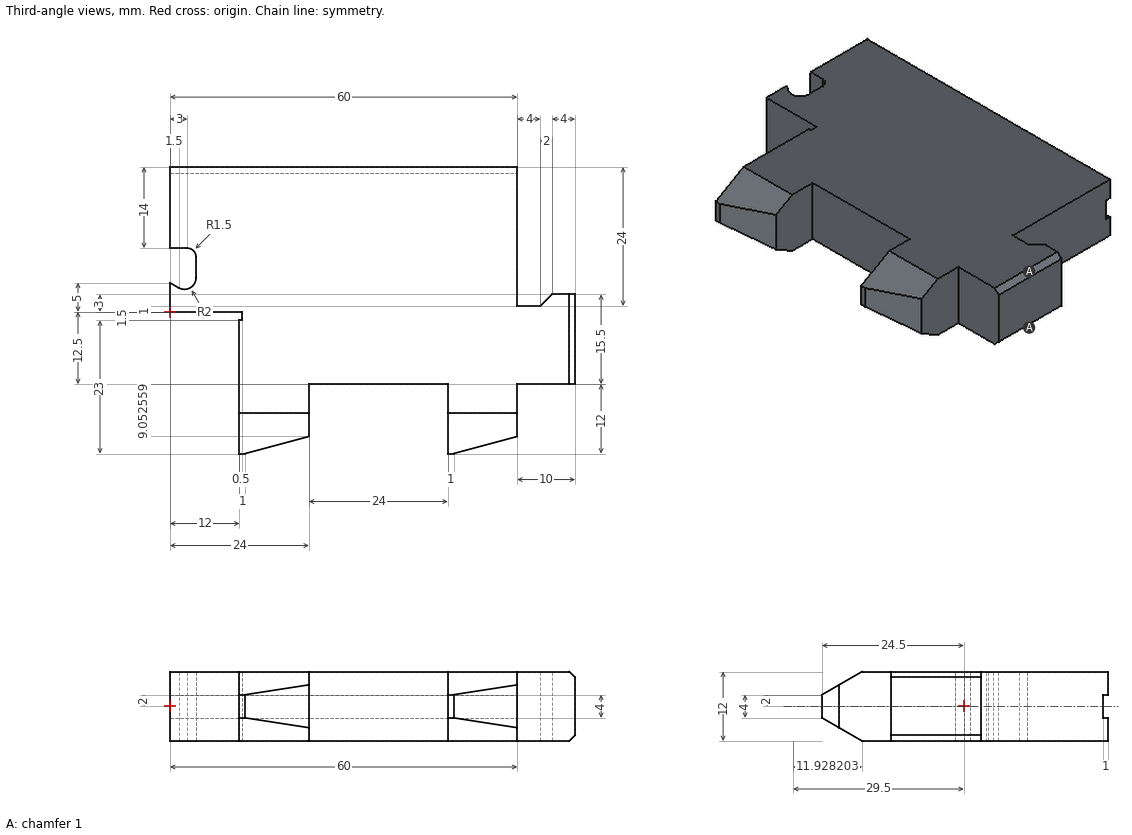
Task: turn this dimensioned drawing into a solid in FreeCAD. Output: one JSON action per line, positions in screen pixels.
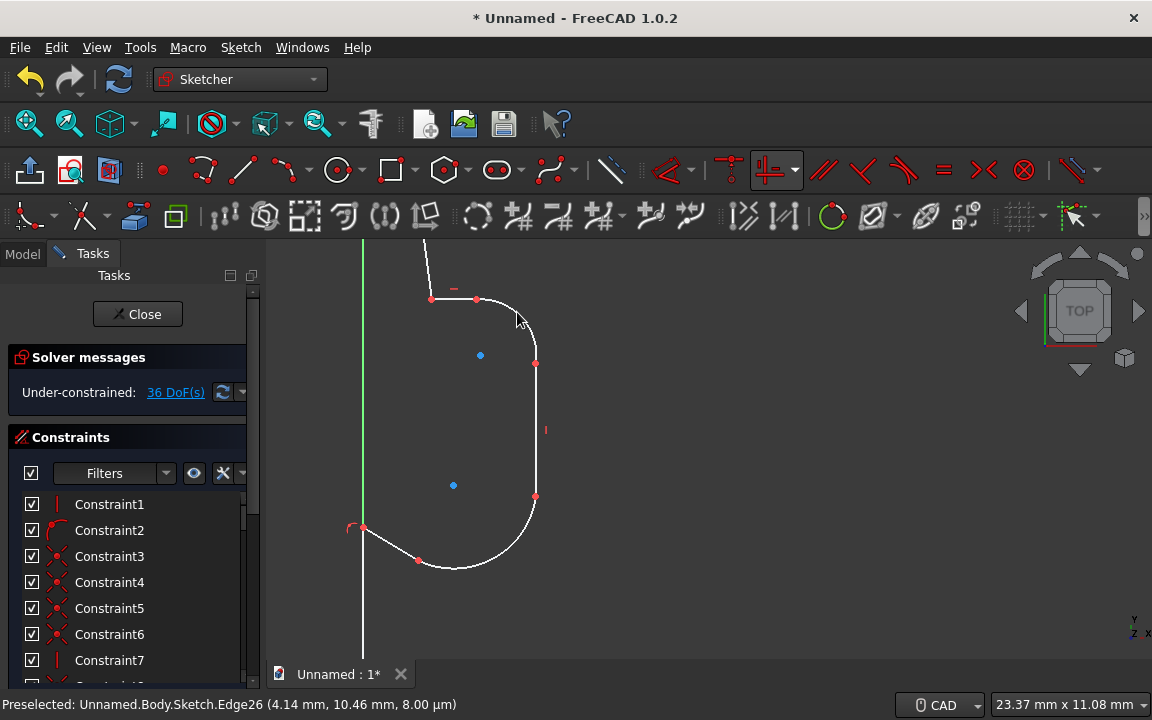
{"action": "scroll", "coordinate": [476, 409], "scroll_direction": "down", "scroll_amount": 10}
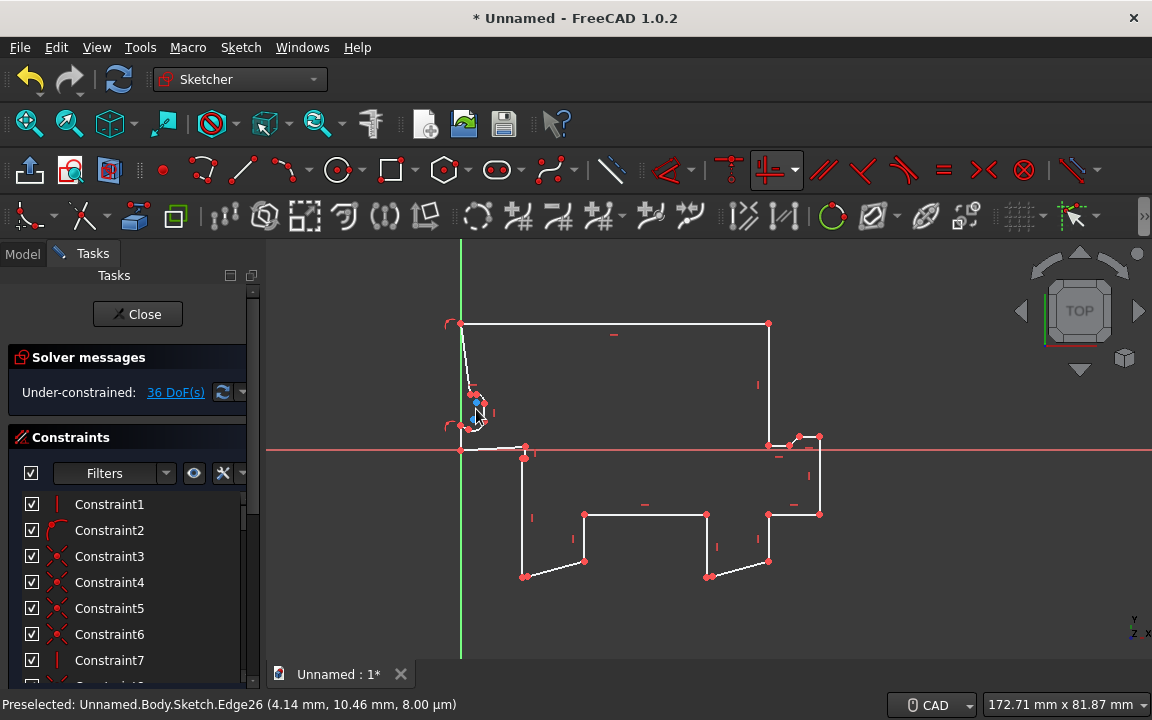
{"action": "scroll", "coordinate": [484, 409], "scroll_direction": "up", "scroll_amount": 5}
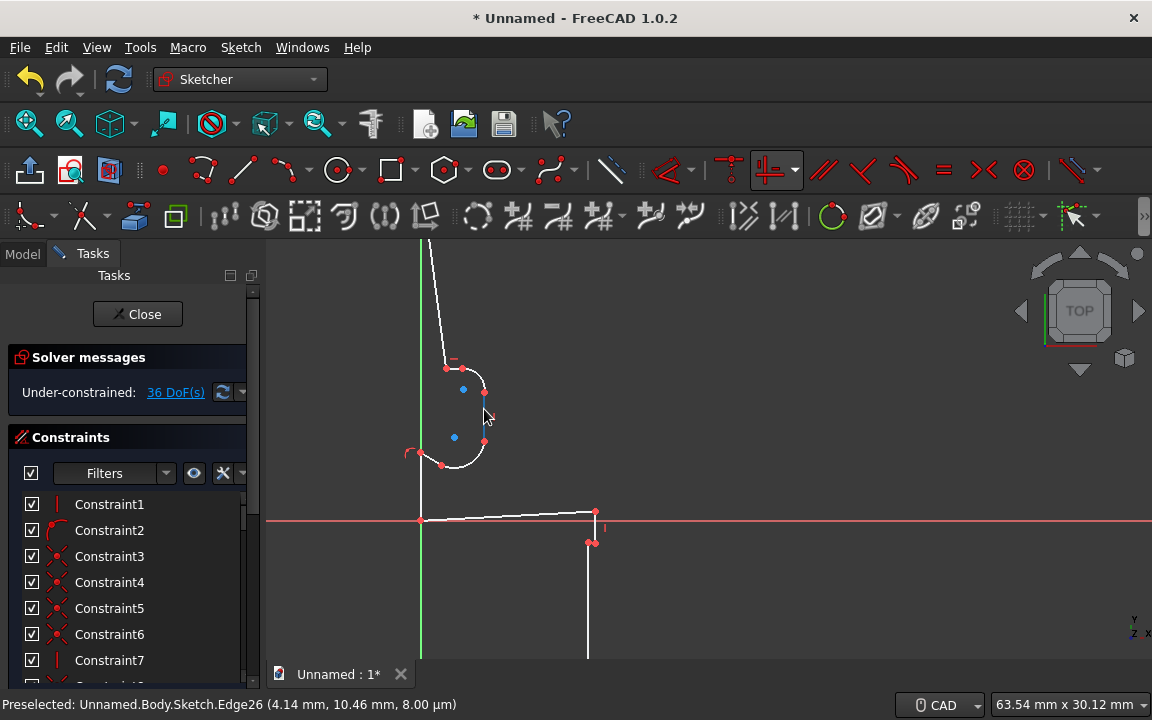
{"action": "left_click", "coordinate": [484, 407]}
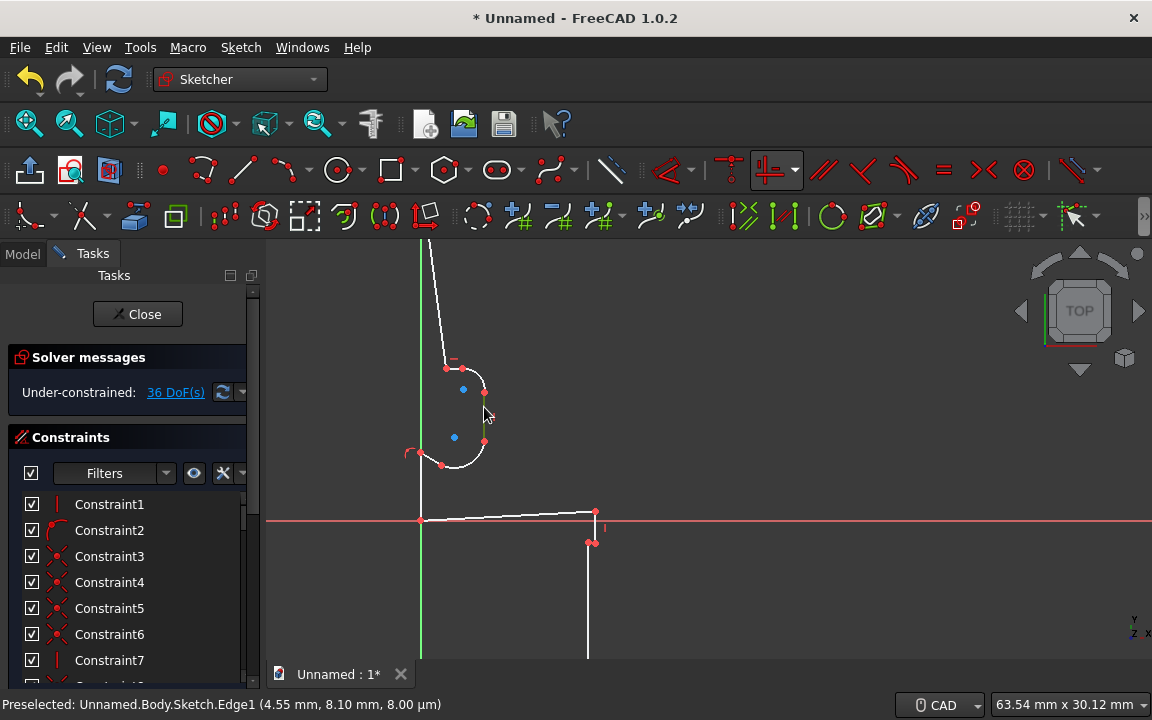
{"action": "left_click", "coordinate": [458, 468]}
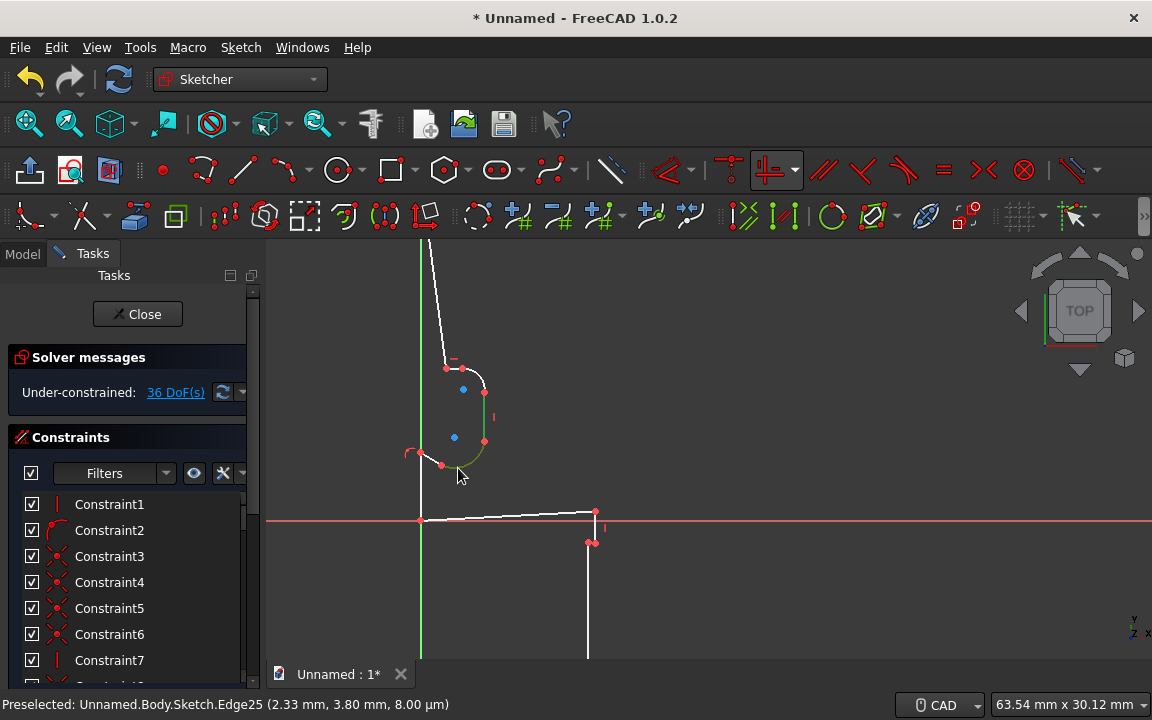
{"action": "left_click", "coordinate": [904, 170]}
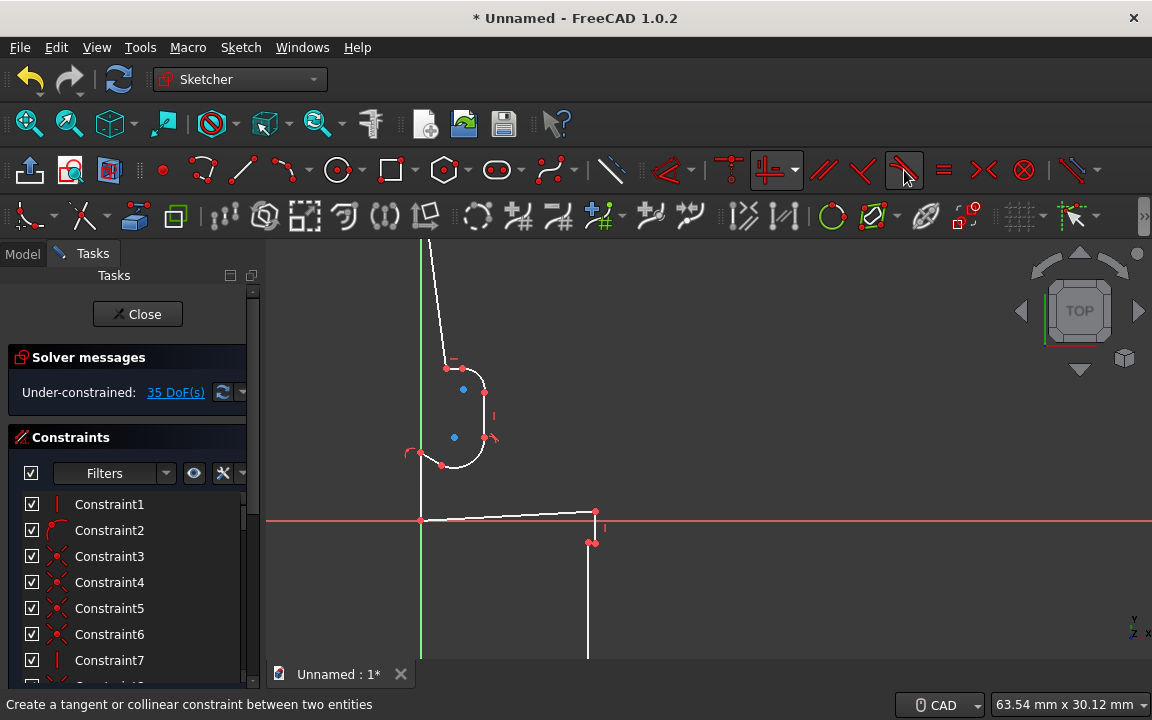
{"action": "left_click", "coordinate": [484, 406]}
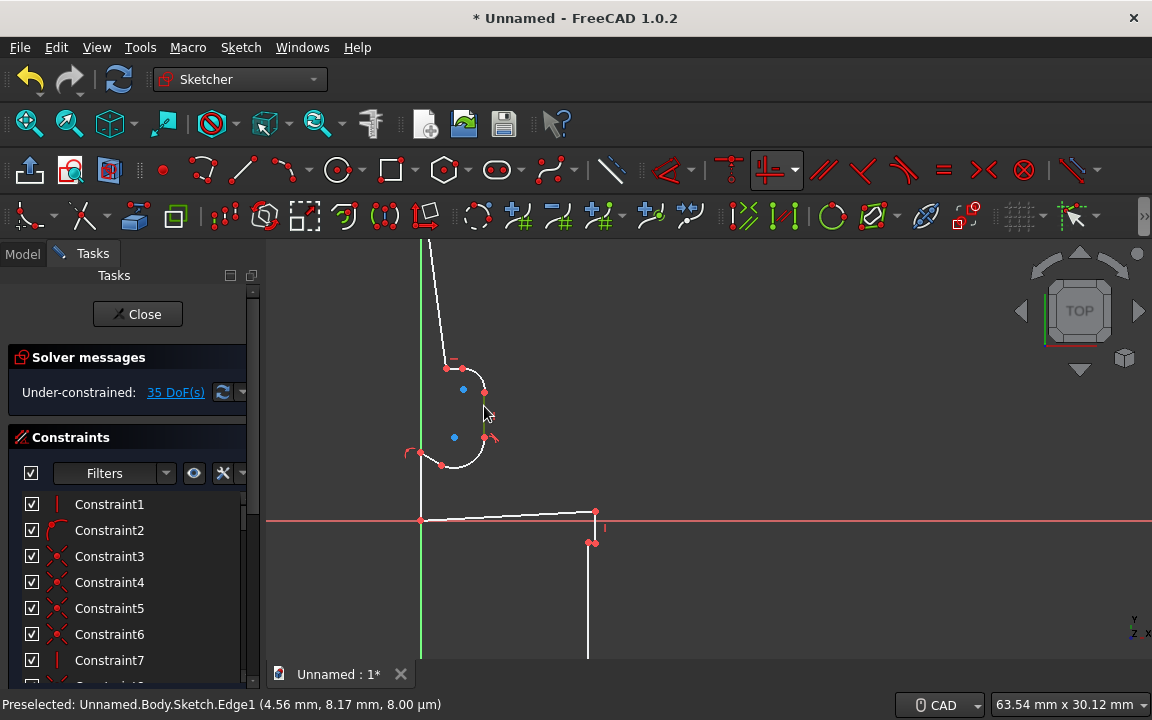
{"action": "scroll", "coordinate": [483, 382], "scroll_direction": "up", "scroll_amount": 2}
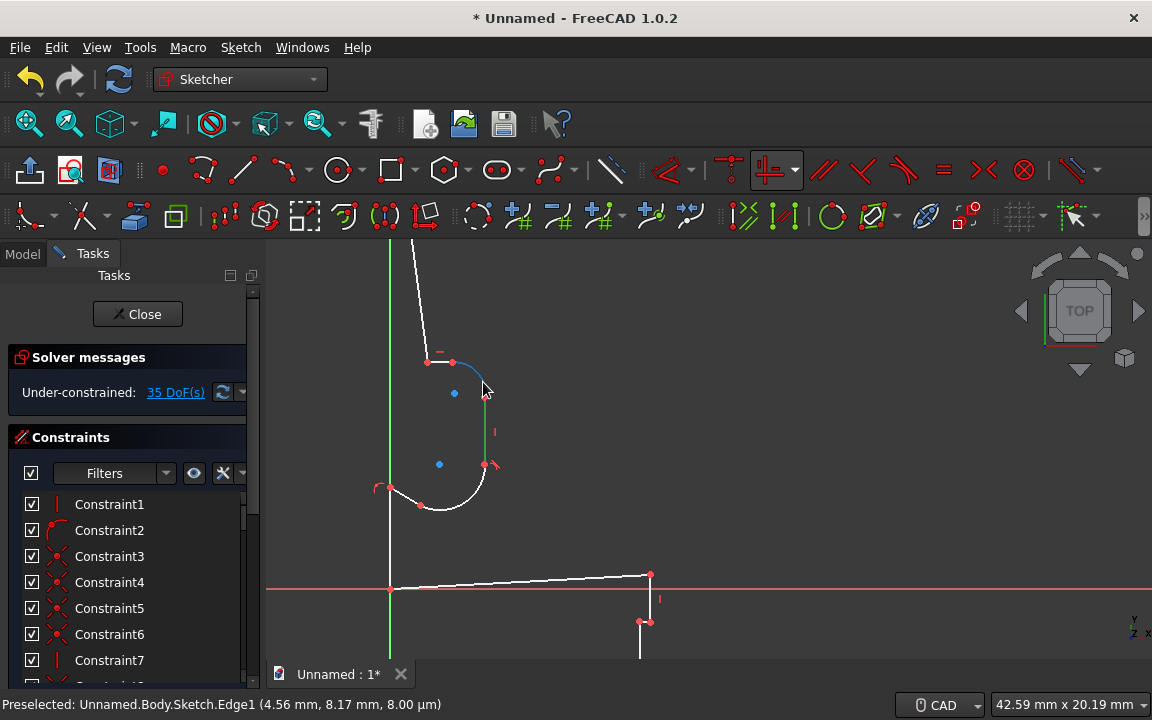
{"action": "left_click", "coordinate": [483, 381]}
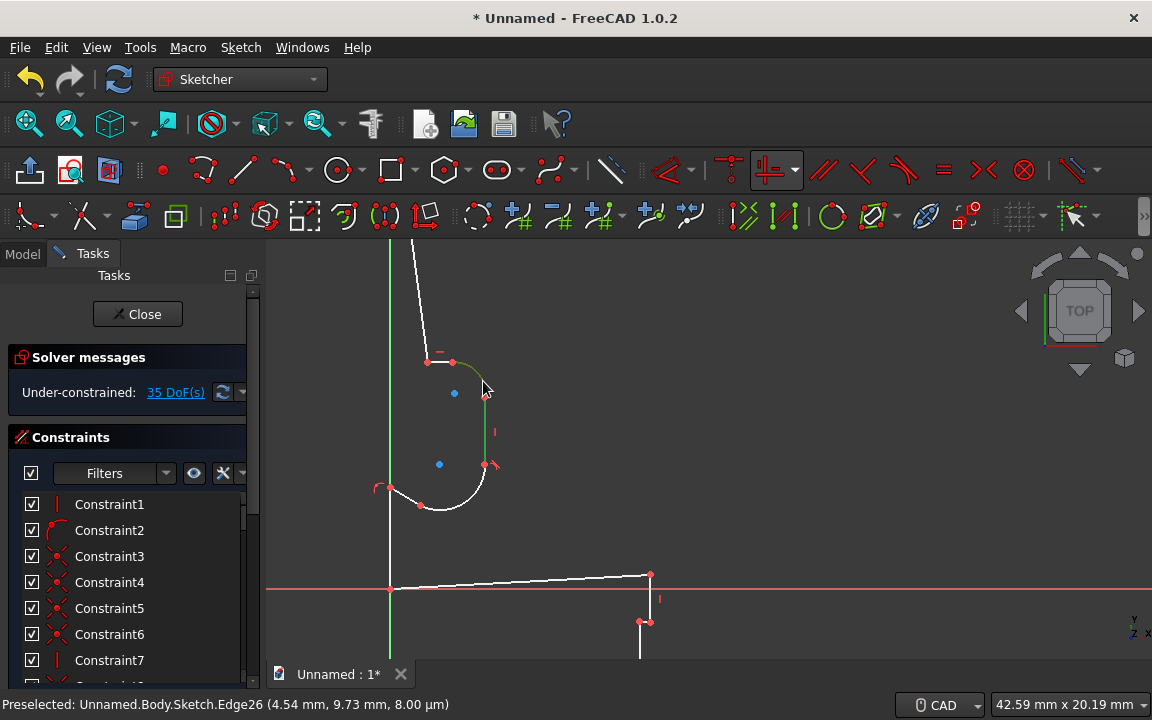
{"action": "left_click", "coordinate": [904, 170]}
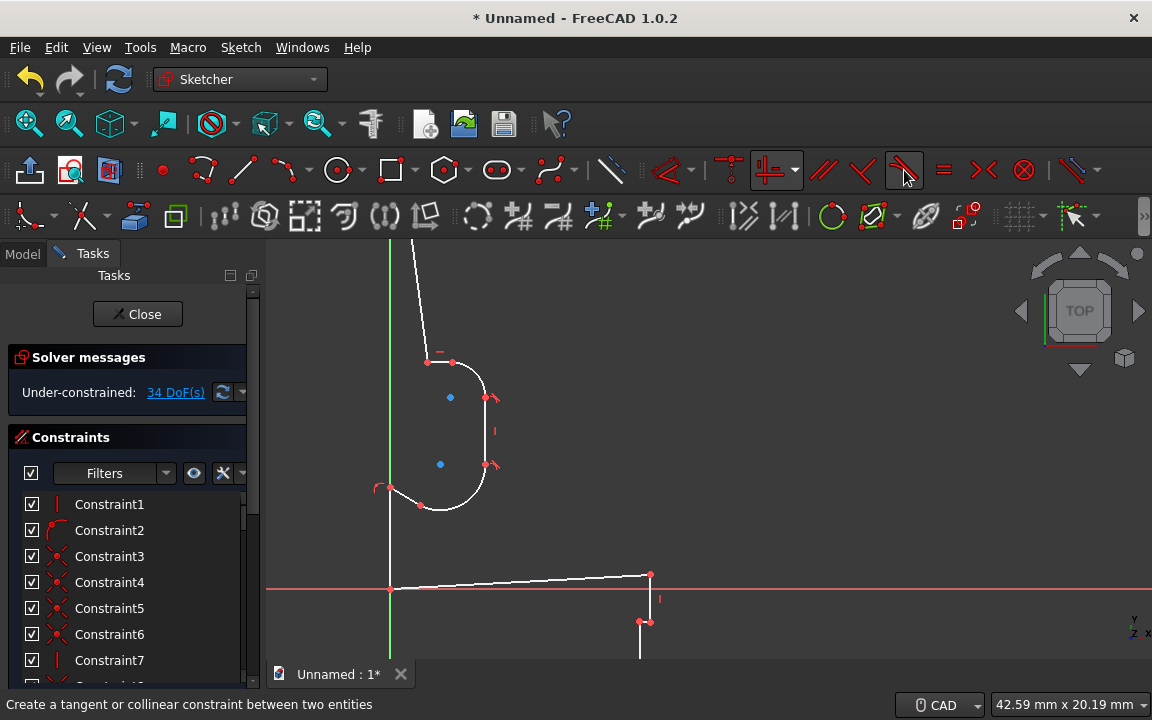
{"action": "scroll", "coordinate": [411, 500], "scroll_direction": "up", "scroll_amount": 2}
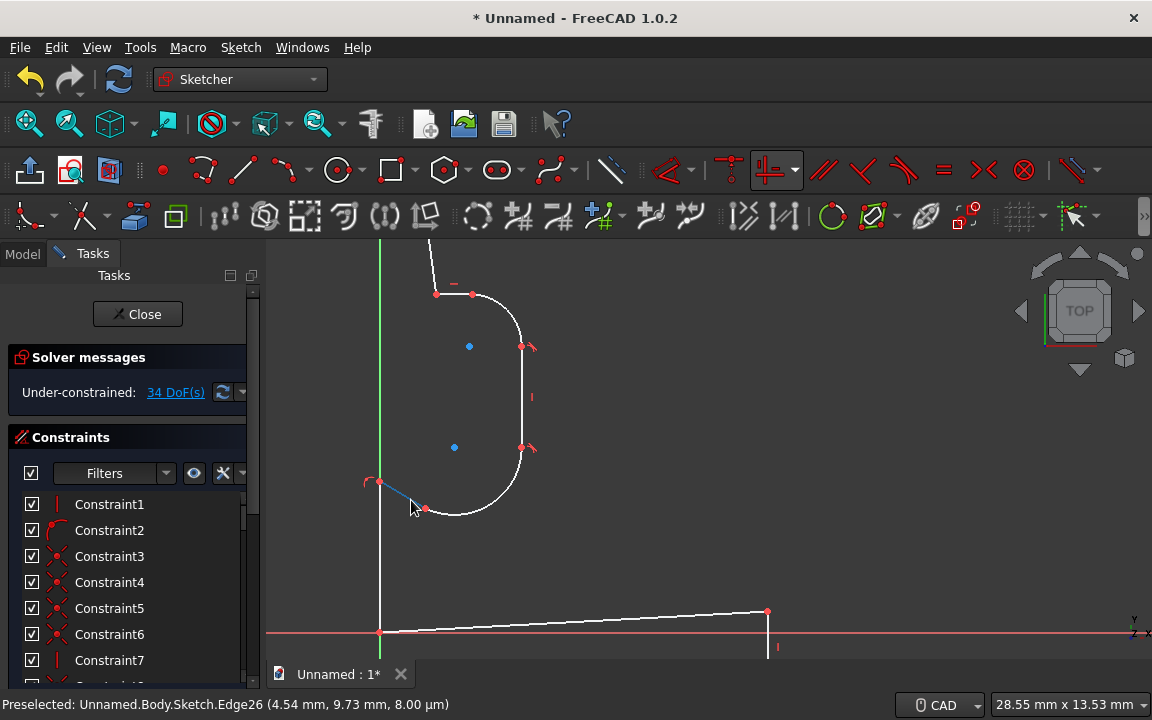
{"action": "left_click", "coordinate": [412, 500]}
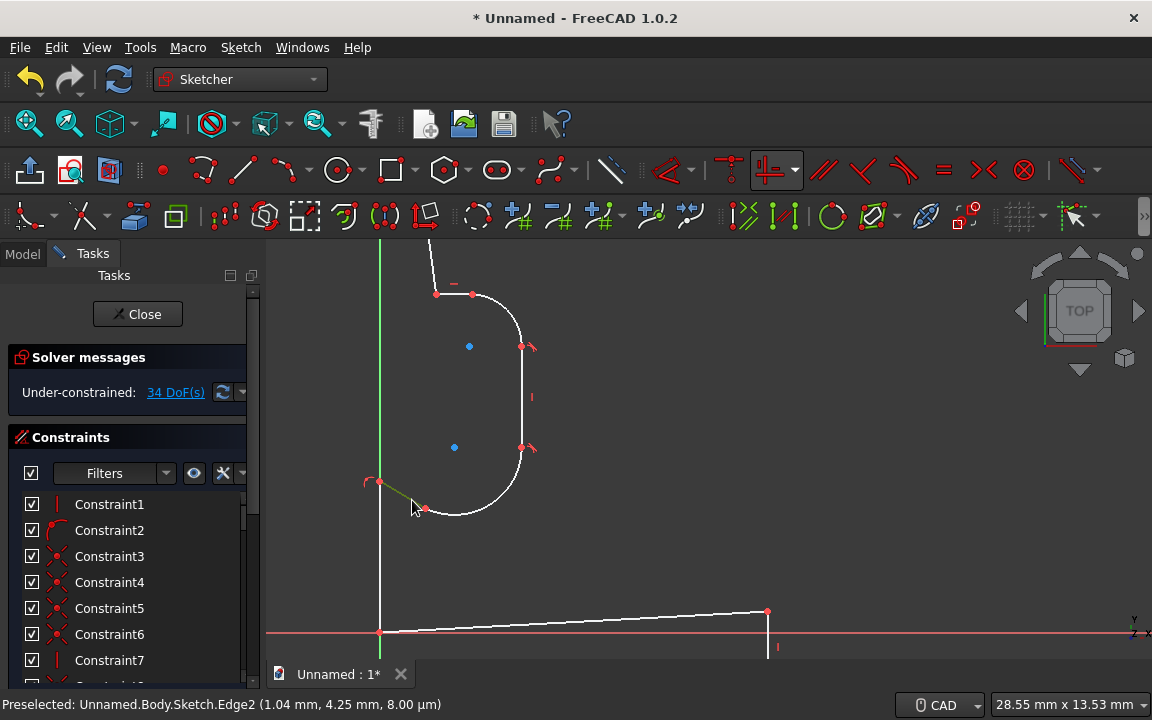
{"action": "scroll", "coordinate": [477, 414], "scroll_direction": "down", "scroll_amount": 9}